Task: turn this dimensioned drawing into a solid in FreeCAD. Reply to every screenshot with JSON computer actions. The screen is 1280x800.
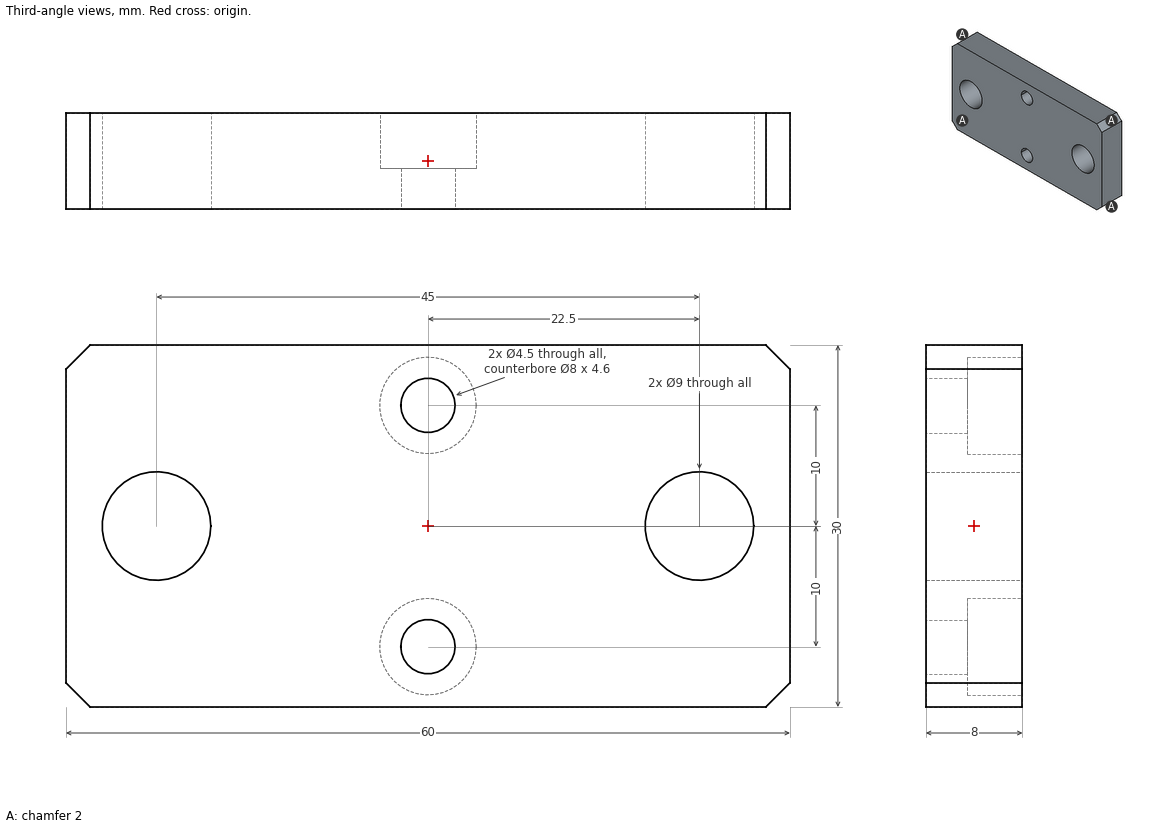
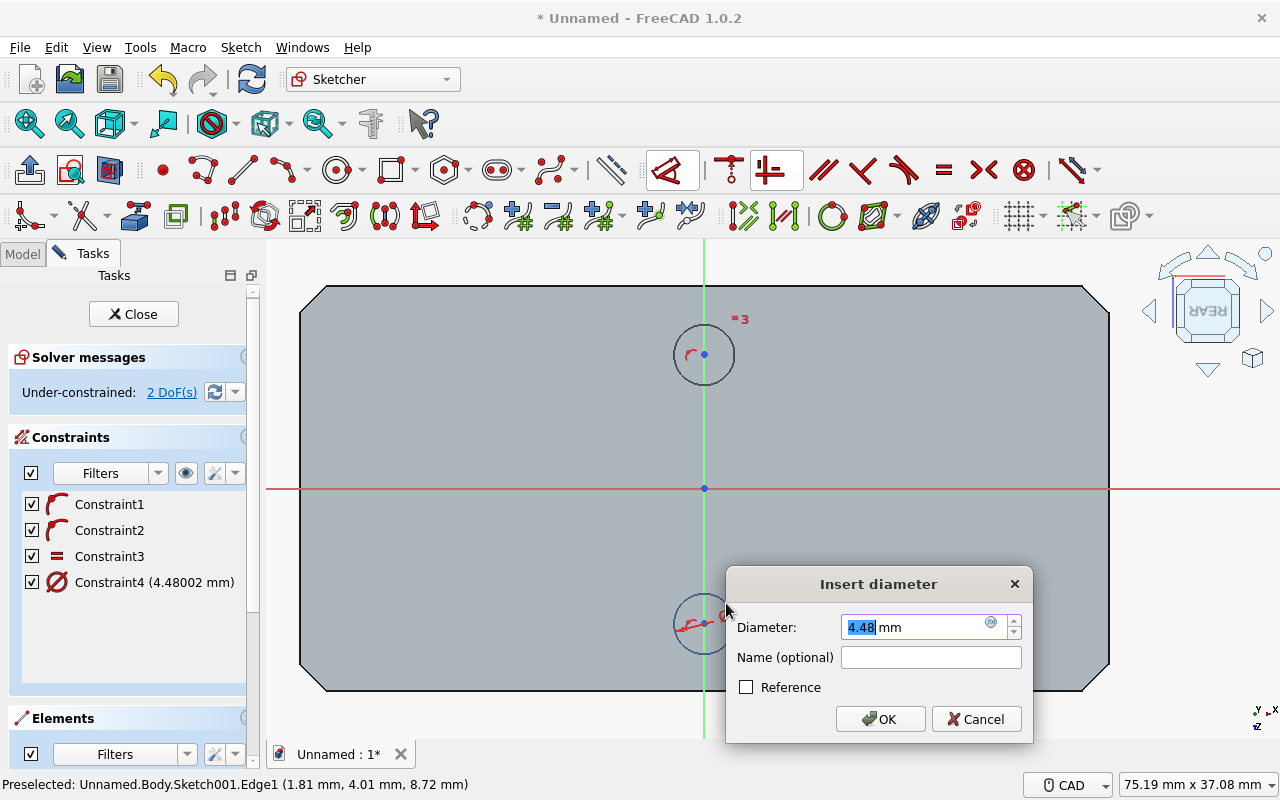
{"action": "type", "text": "4.5"}
{"action": "key", "text": "Return"}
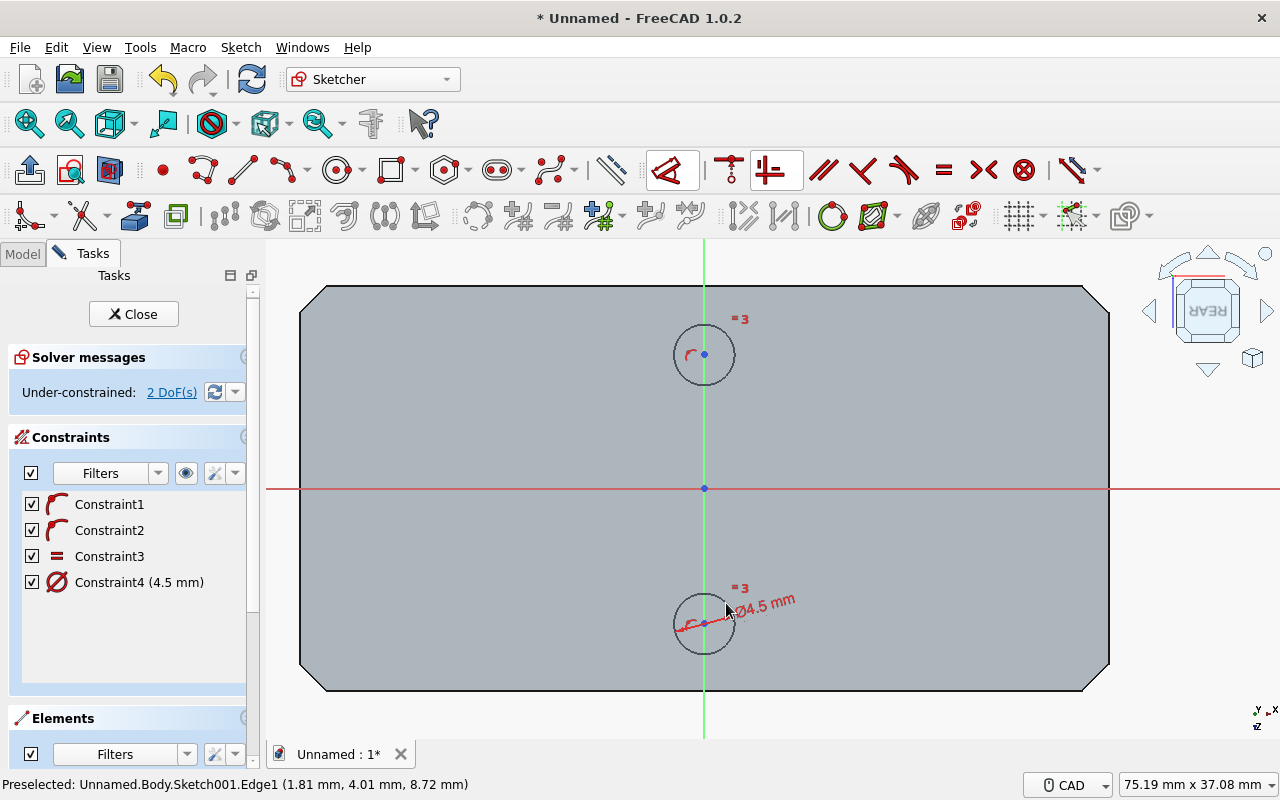
{"action": "left_click", "coordinate": [704, 624]}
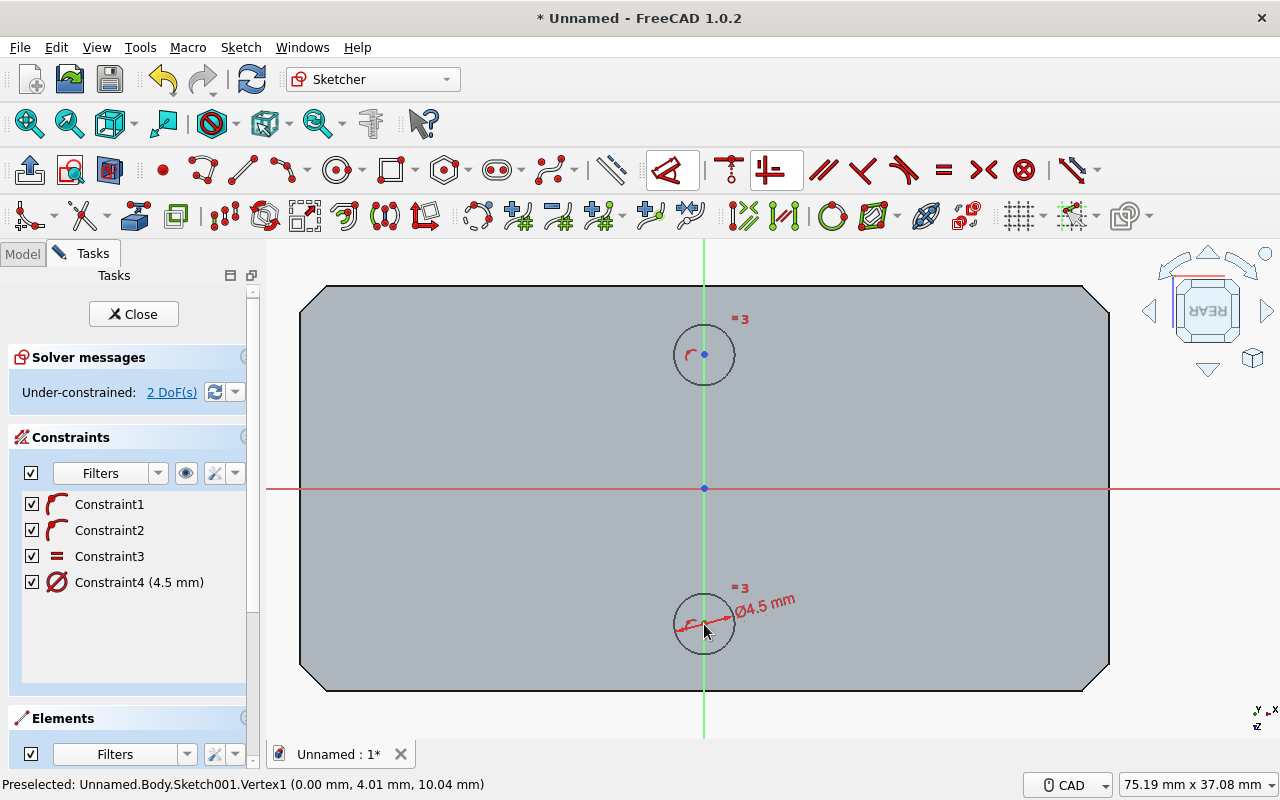
{"action": "left_click", "coordinate": [694, 170]}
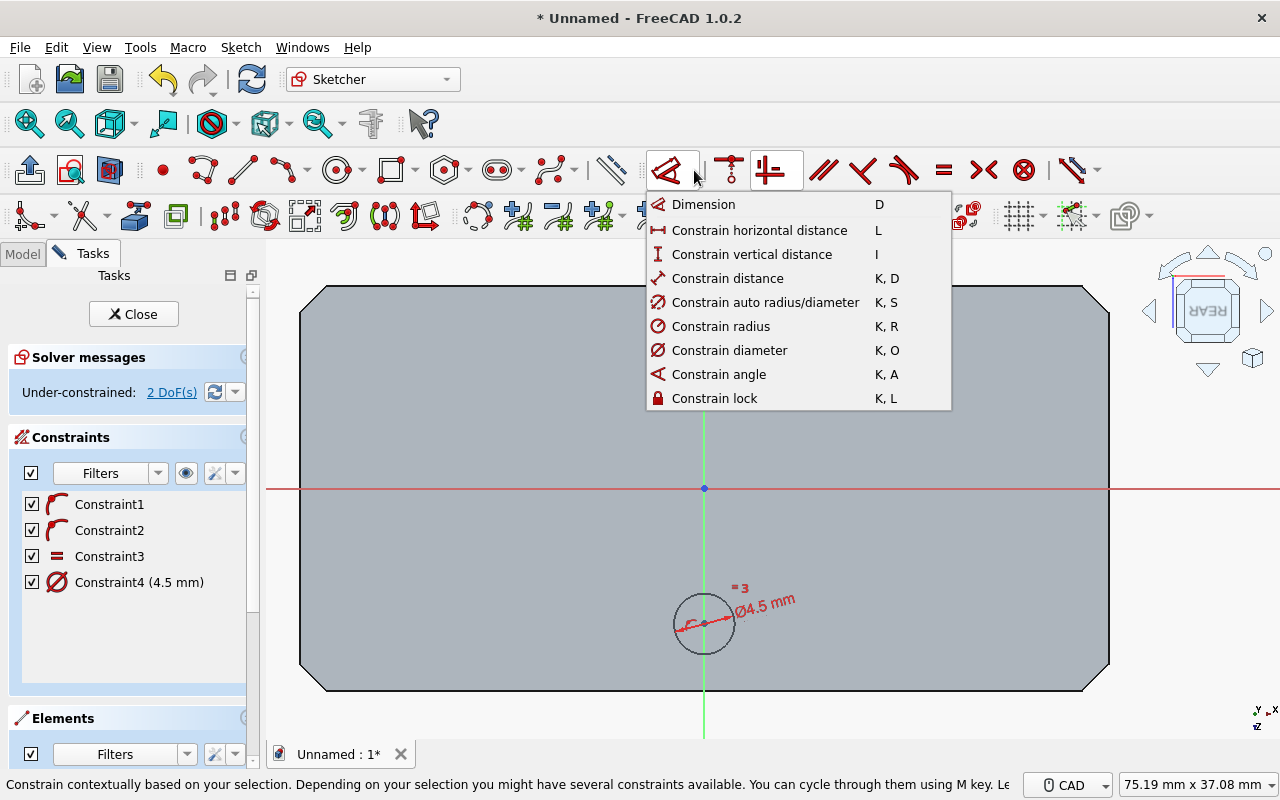
{"action": "left_click", "coordinate": [799, 254]}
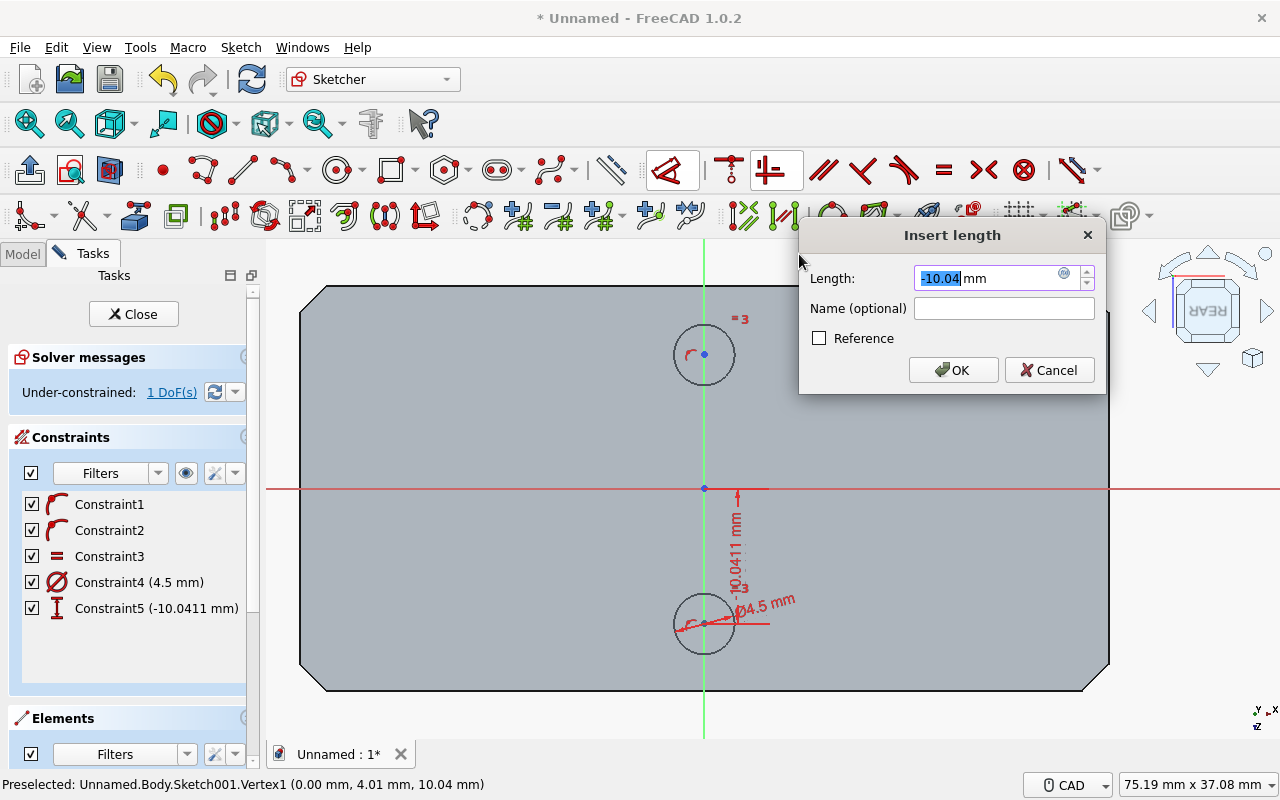
{"action": "type", "text": "-10"}
{"action": "key", "text": "Return"}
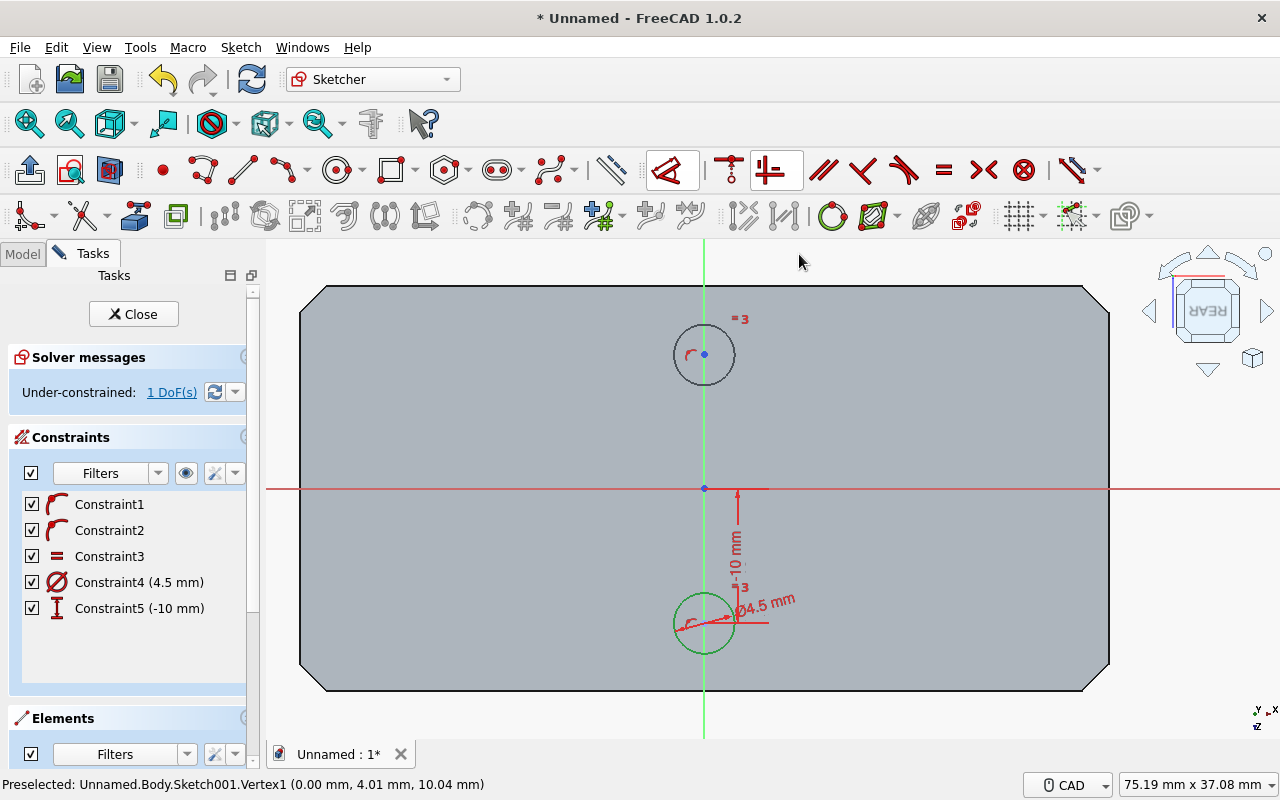
{"action": "left_click", "coordinate": [704, 355]}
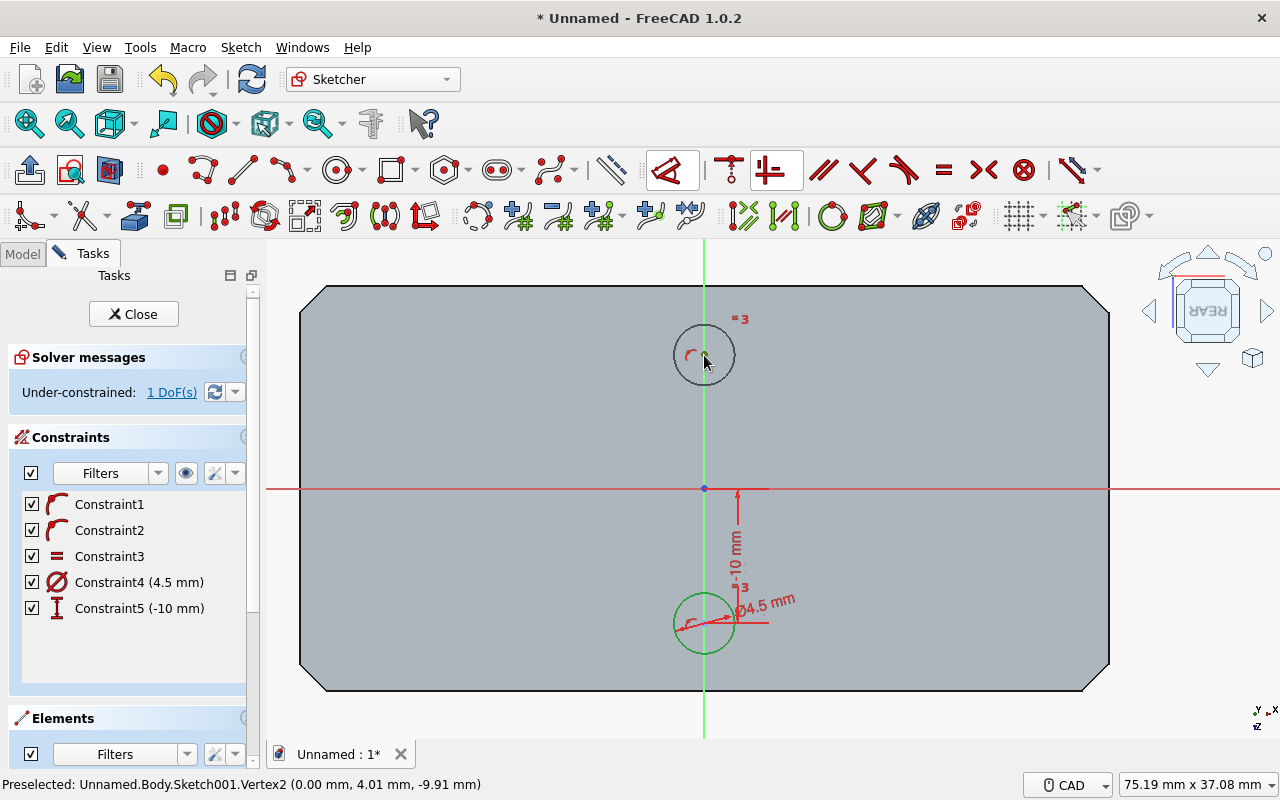
{"action": "left_click", "coordinate": [694, 170]}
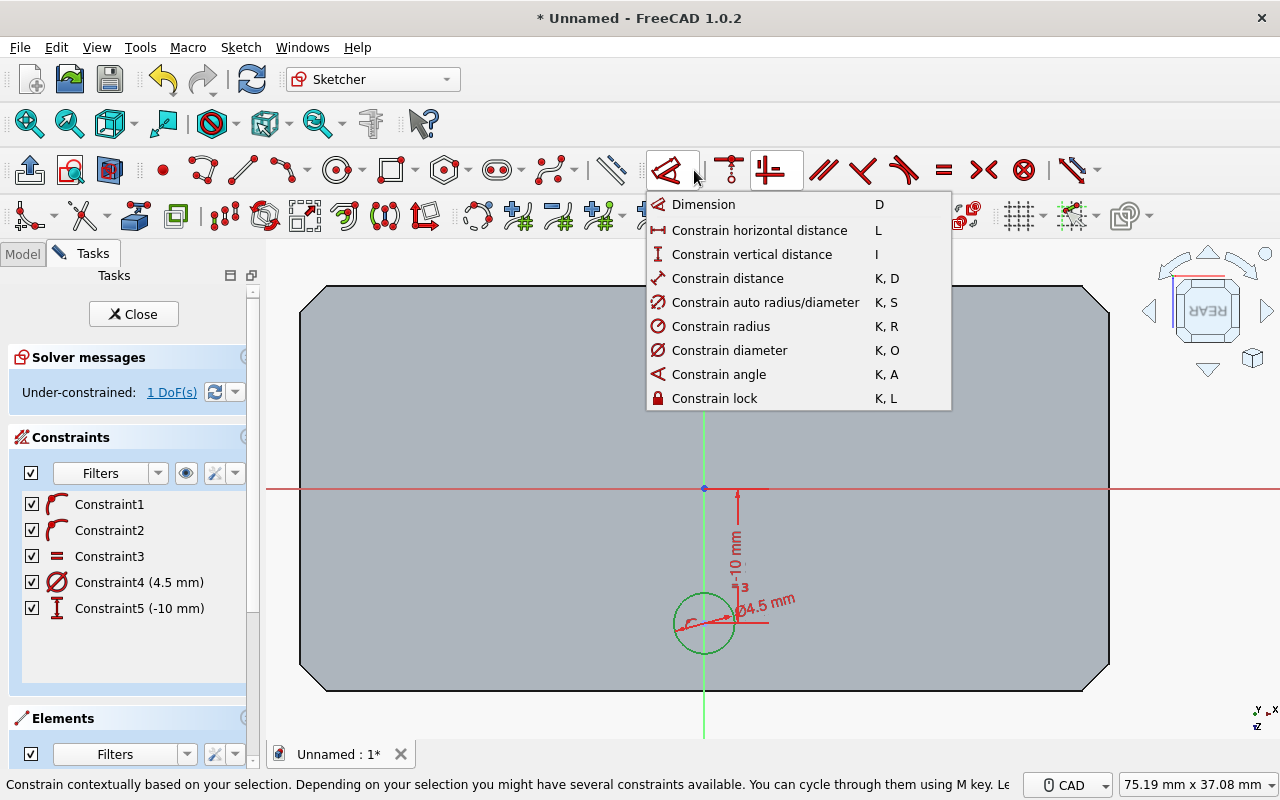
{"action": "left_click", "coordinate": [799, 254]}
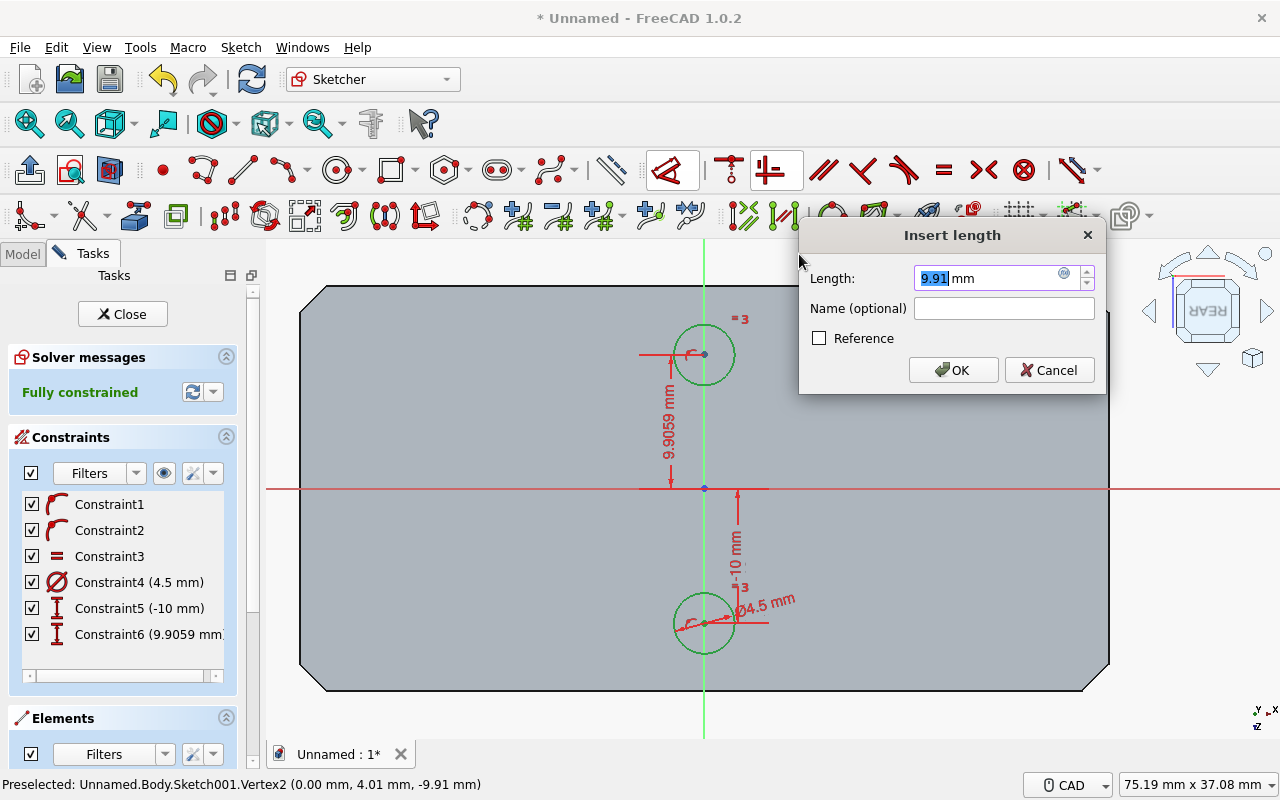
{"action": "type", "text": "10"}
{"action": "key", "text": "Return"}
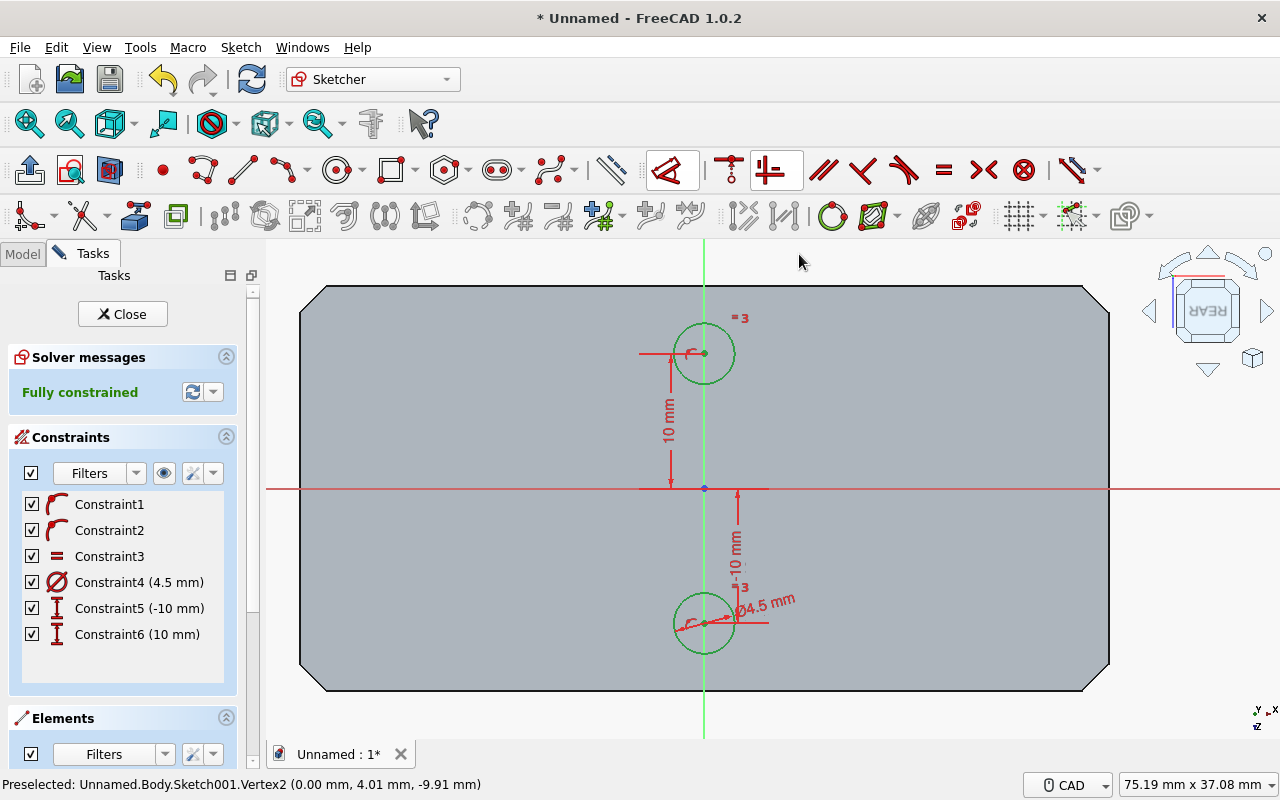
{"action": "left_click", "coordinate": [123, 314]}